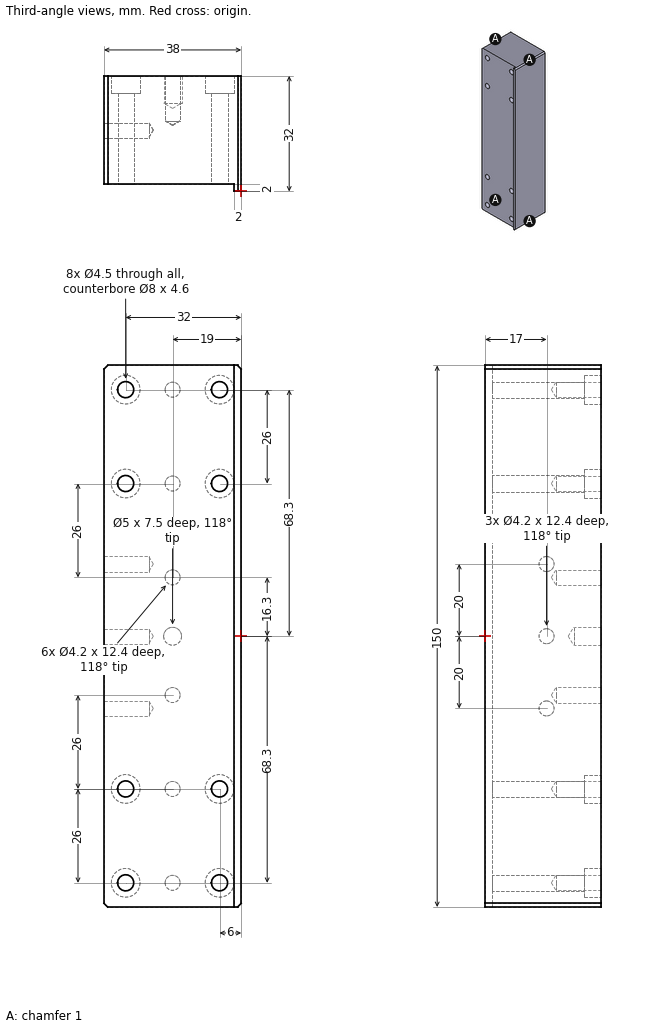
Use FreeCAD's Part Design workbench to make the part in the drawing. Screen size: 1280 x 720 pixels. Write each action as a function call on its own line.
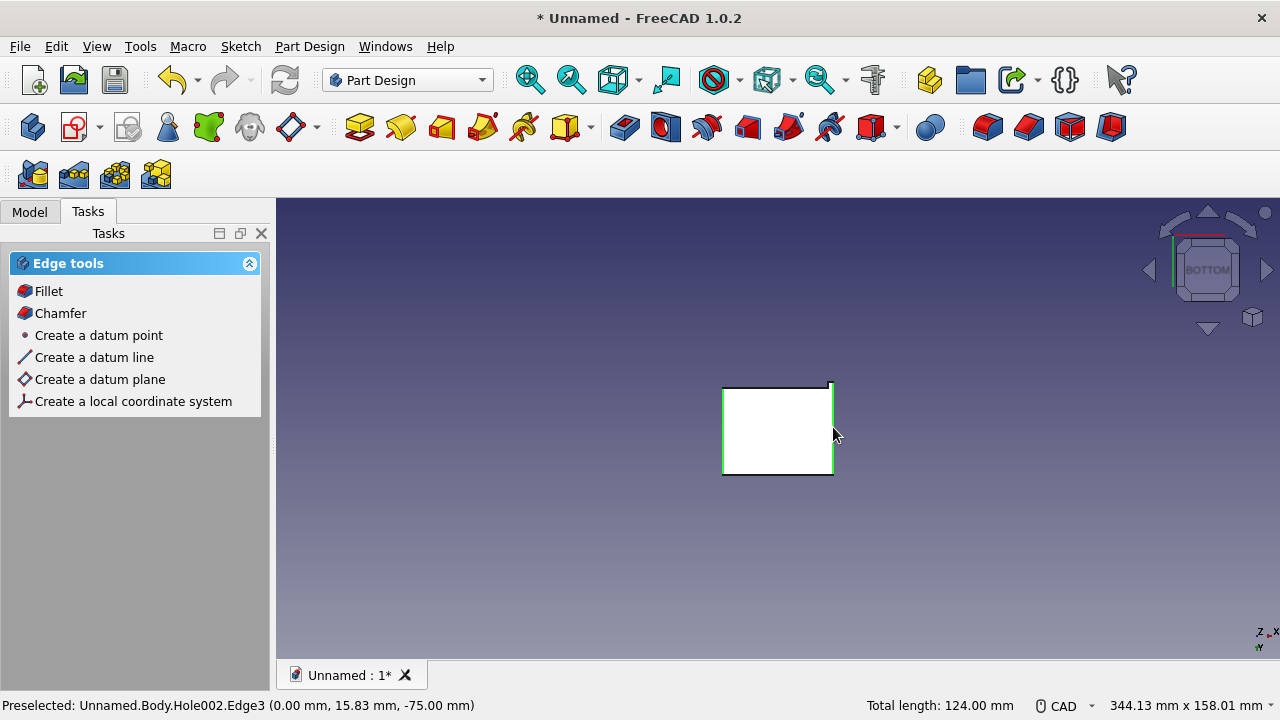
click(1029, 128)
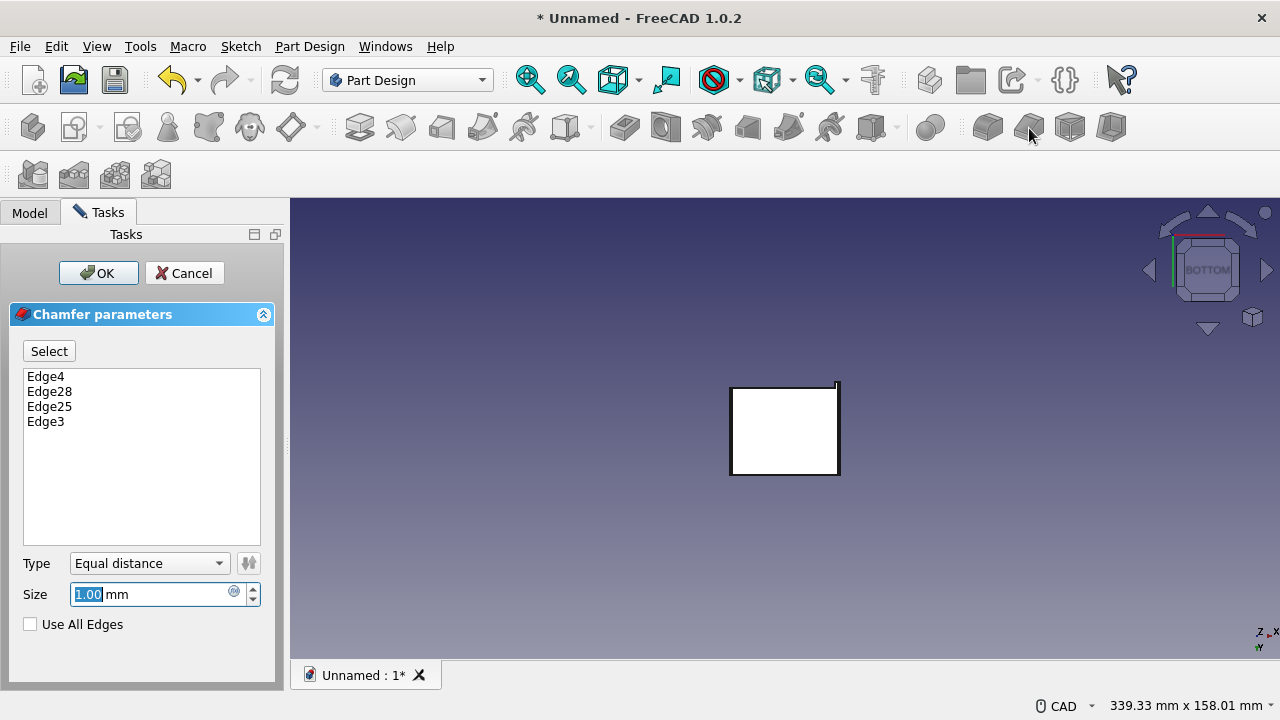
text(1)
key(Tab)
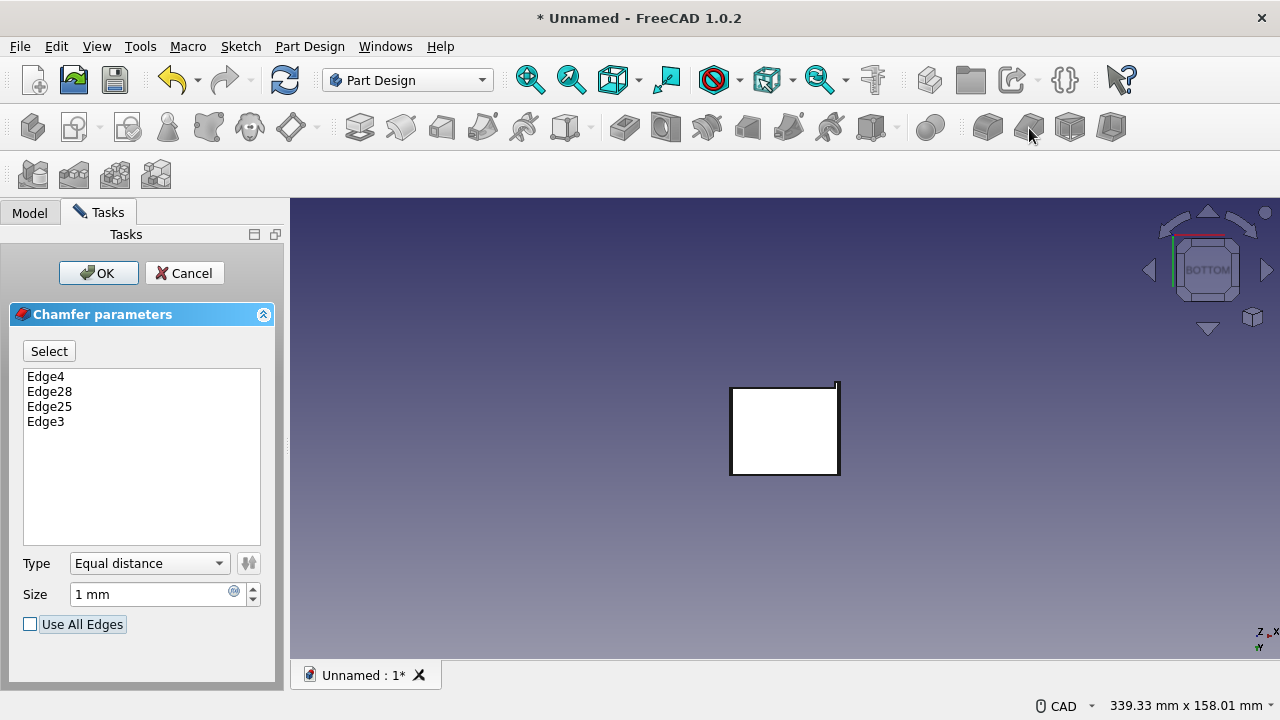
click(99, 273)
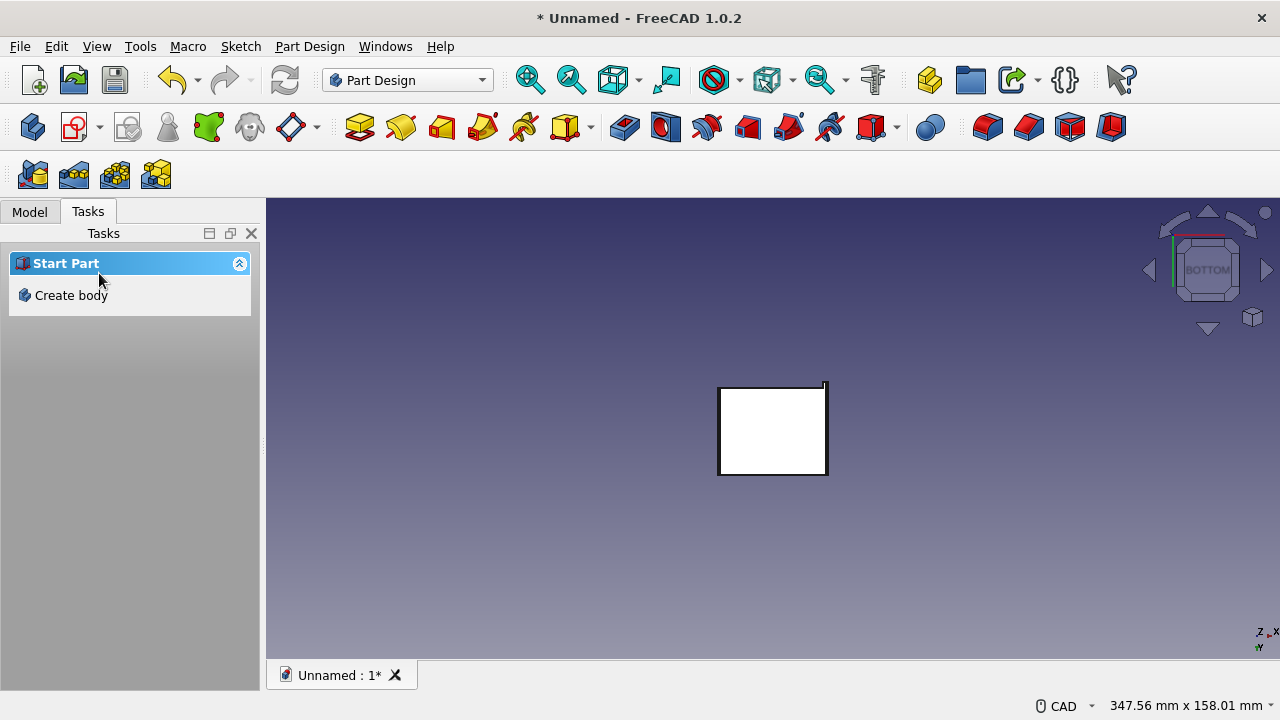
click(531, 80)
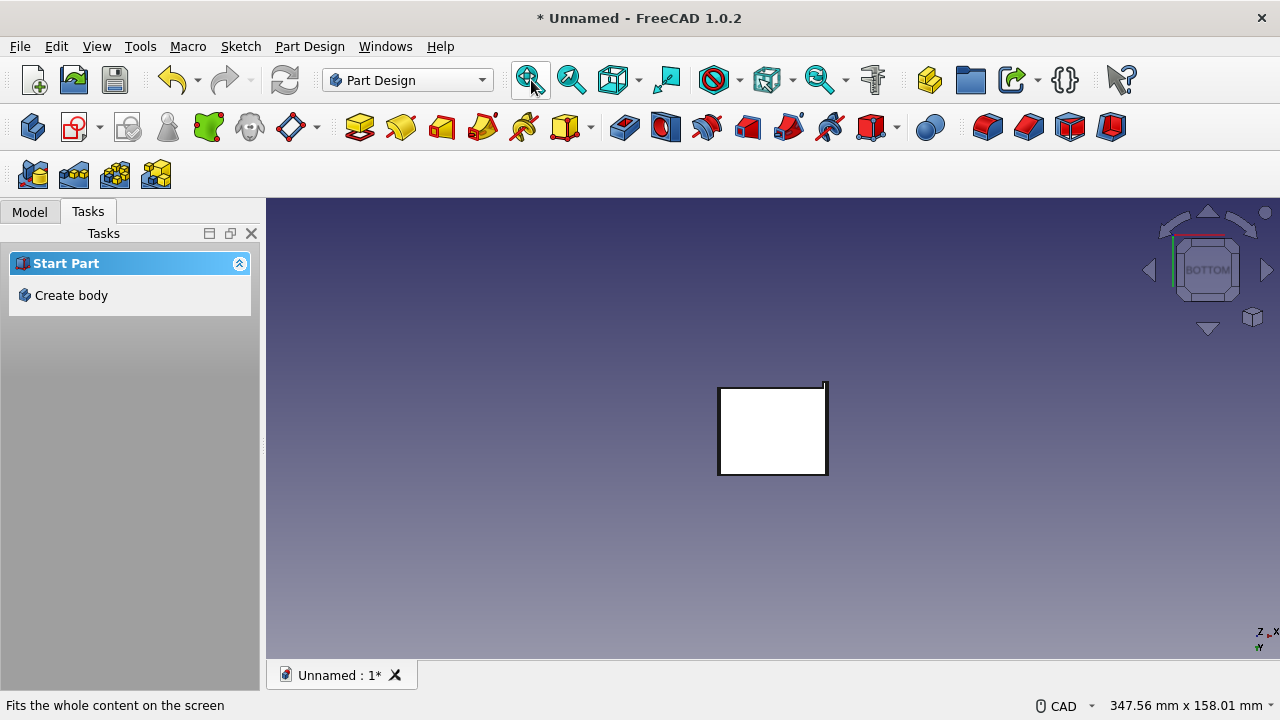
key(4)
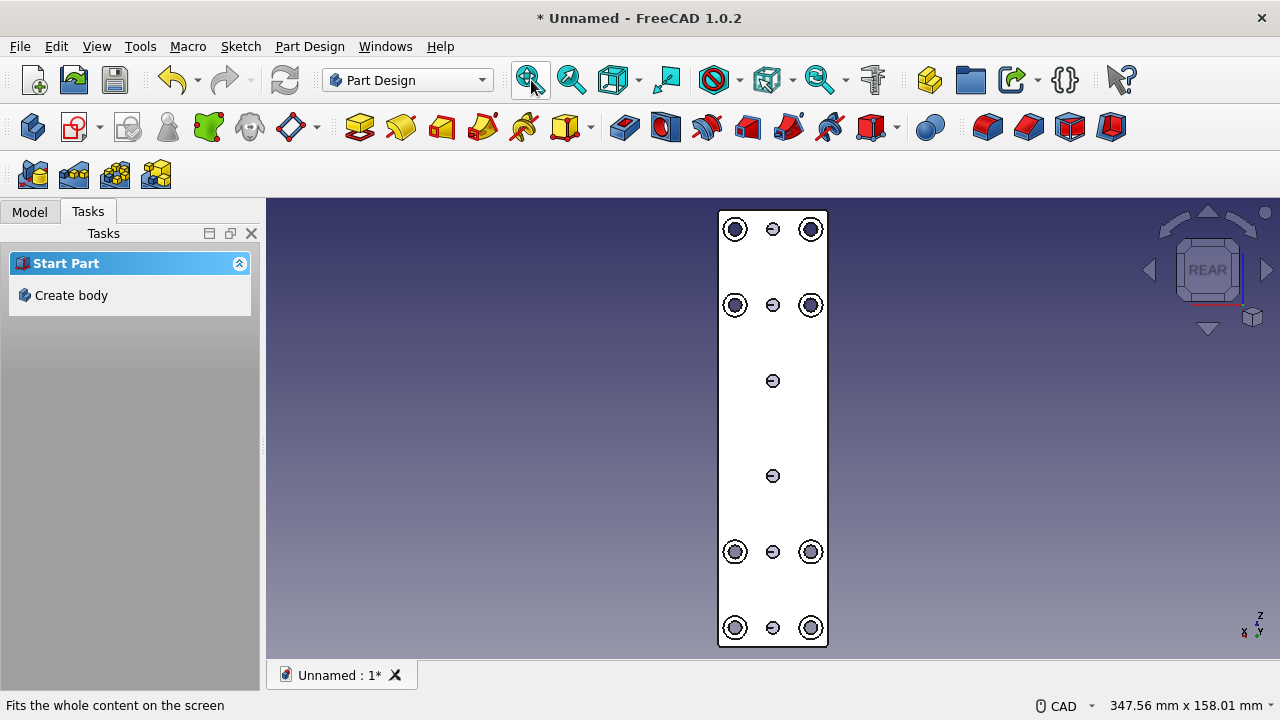
click(773, 427)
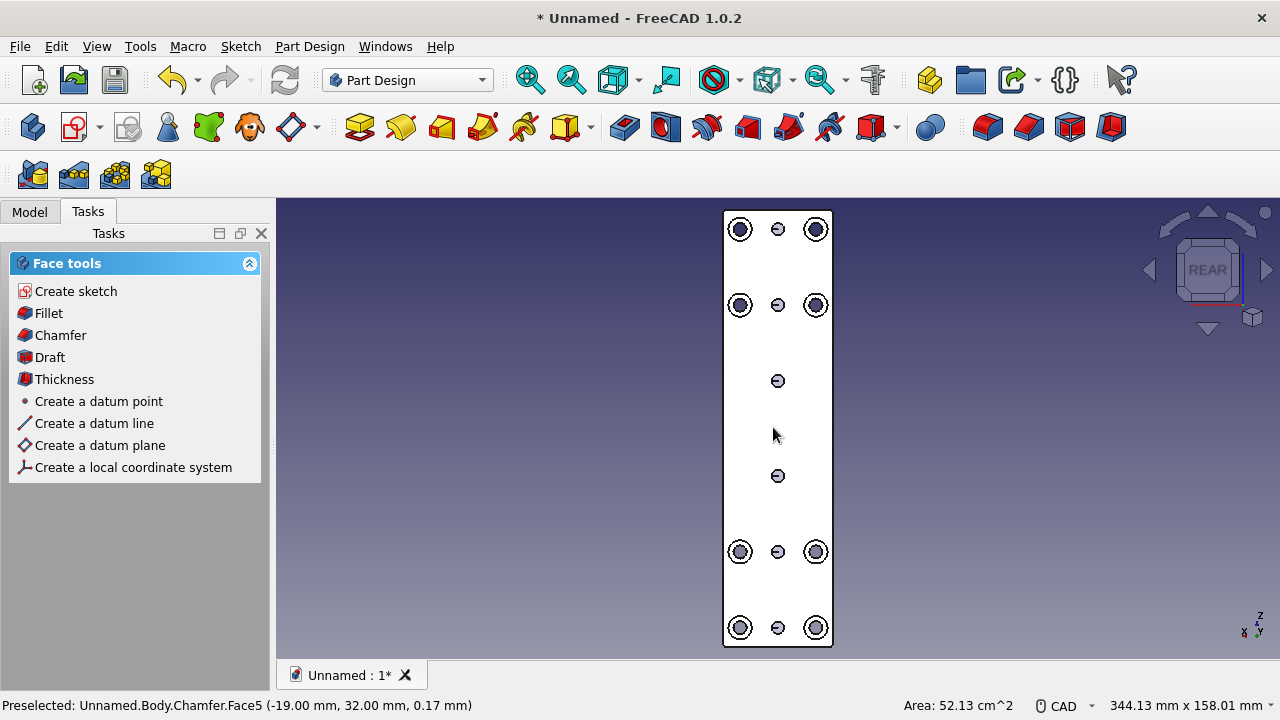
click(74, 128)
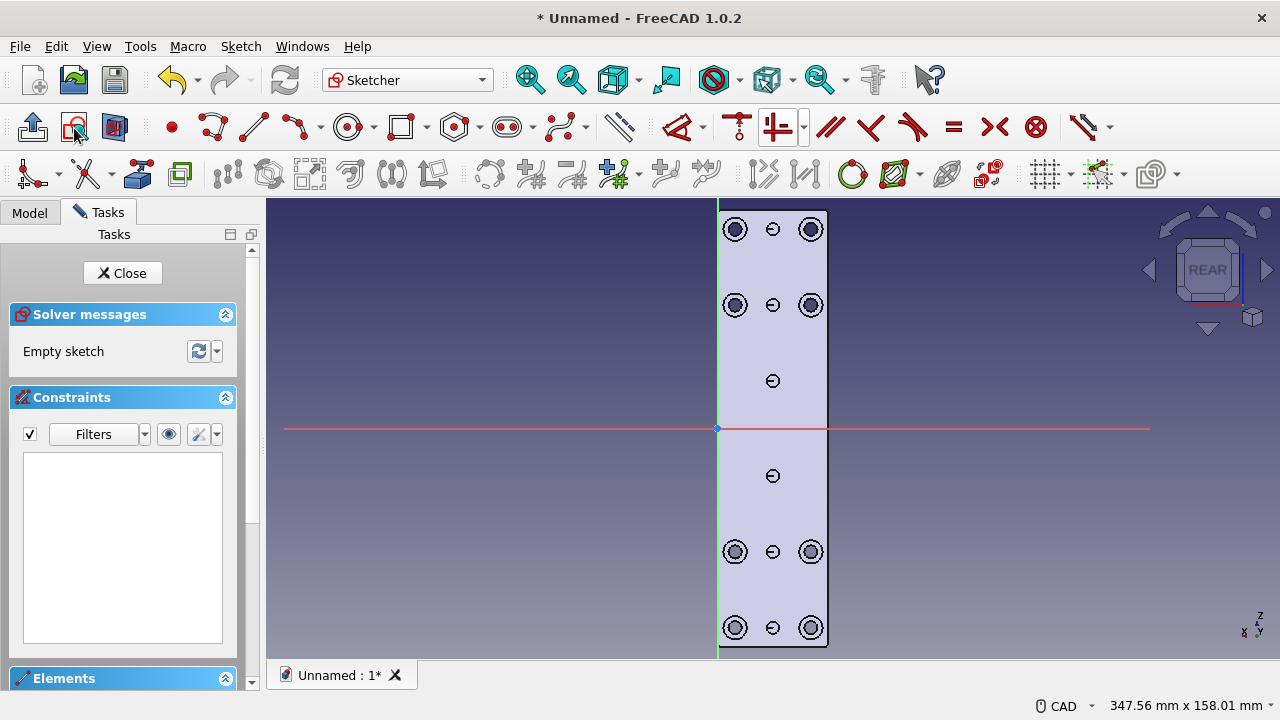
scroll(777, 428, up, 15)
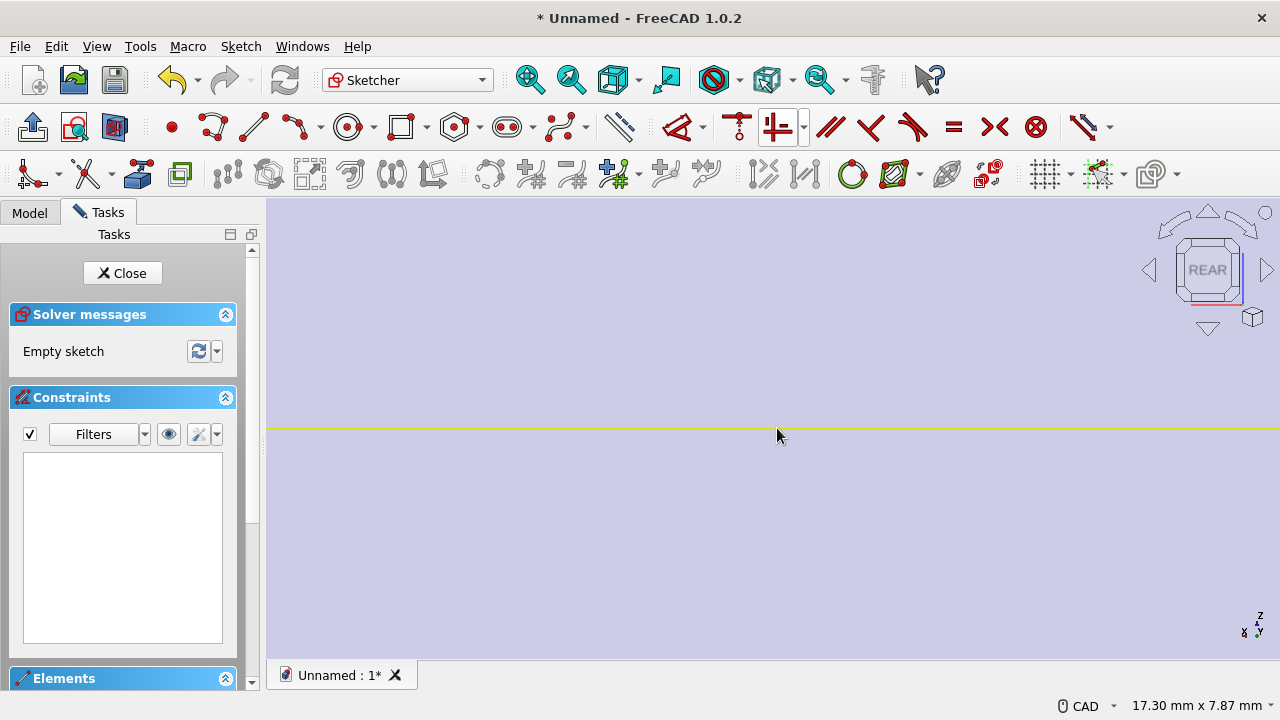
click(348, 128)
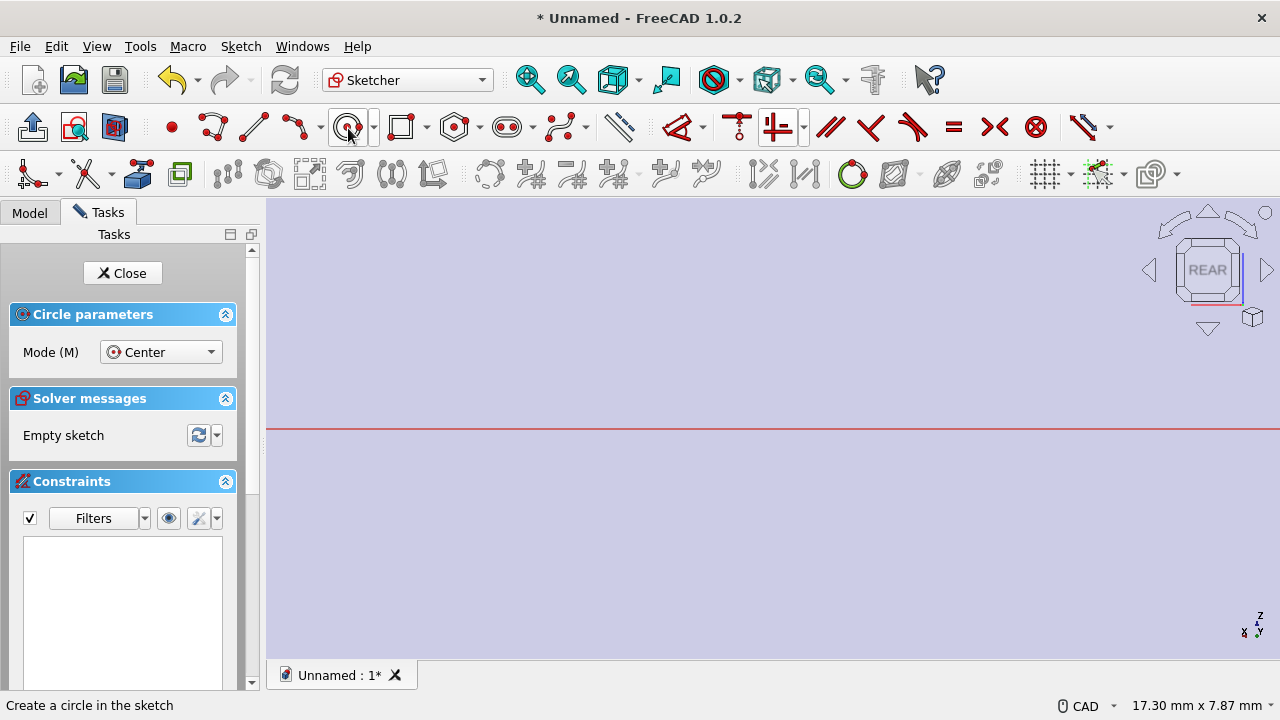
click(687, 428)
move(791, 325)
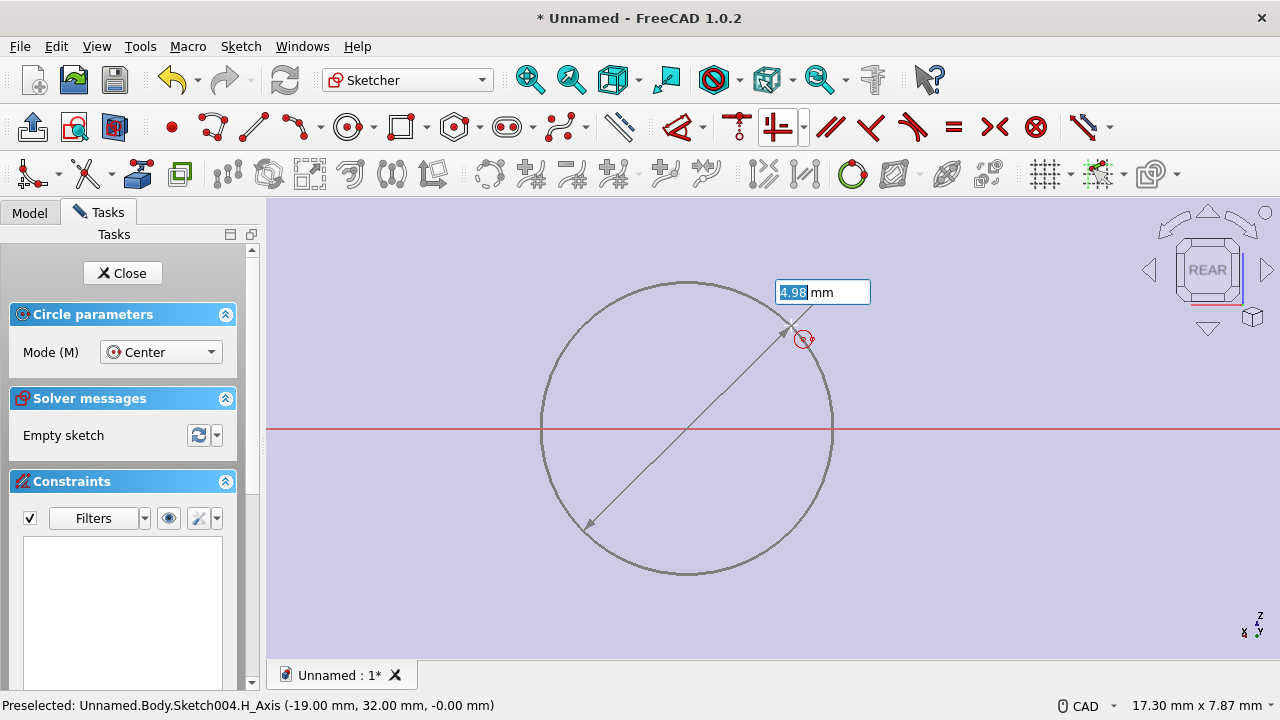
text(5)
key(Return)
key(Escape)